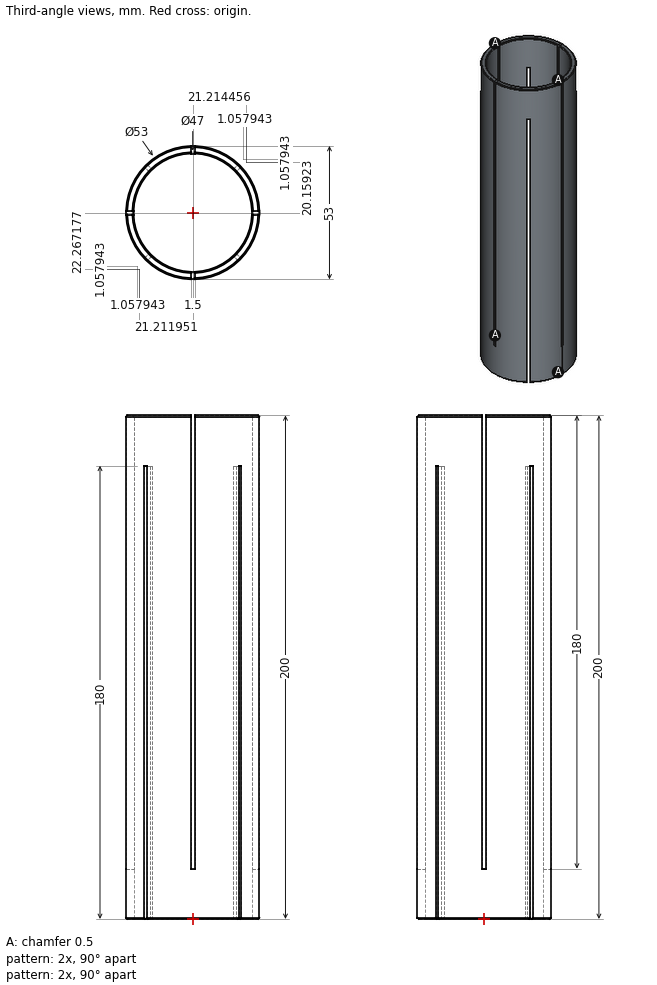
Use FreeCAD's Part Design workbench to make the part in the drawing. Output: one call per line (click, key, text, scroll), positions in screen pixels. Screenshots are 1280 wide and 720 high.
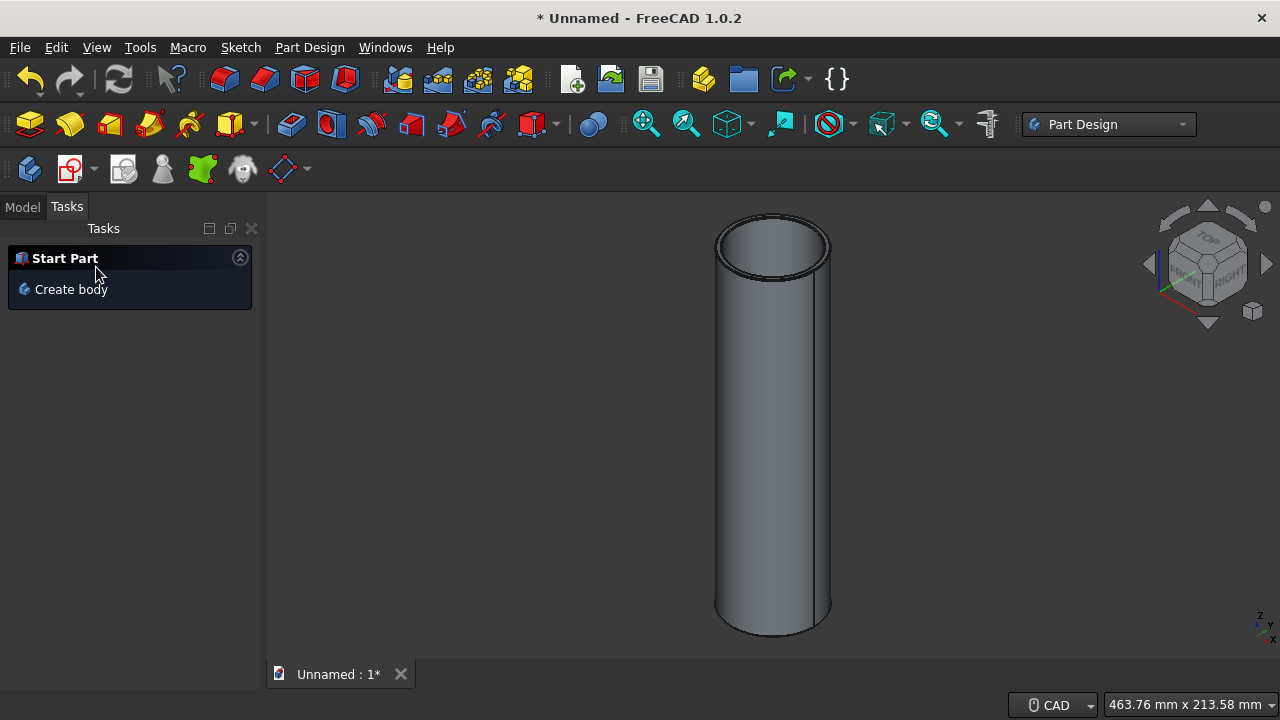
scroll(719, 238, up, 11)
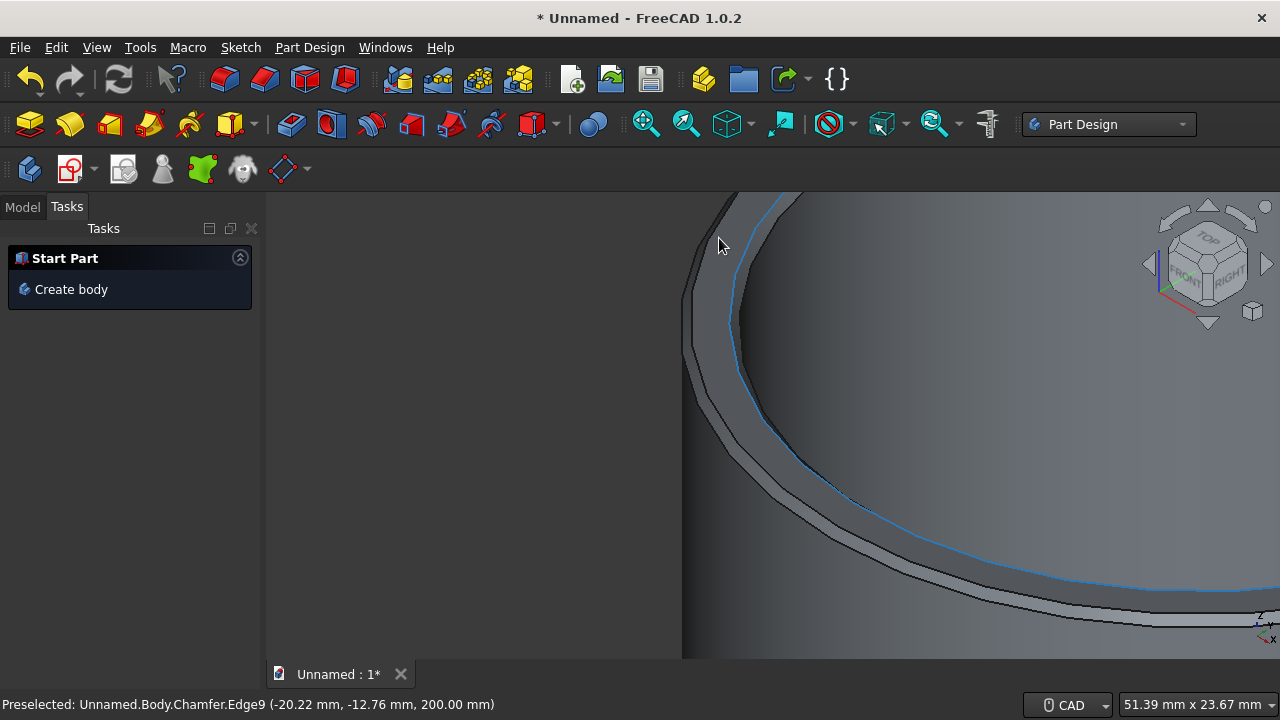
click(719, 245)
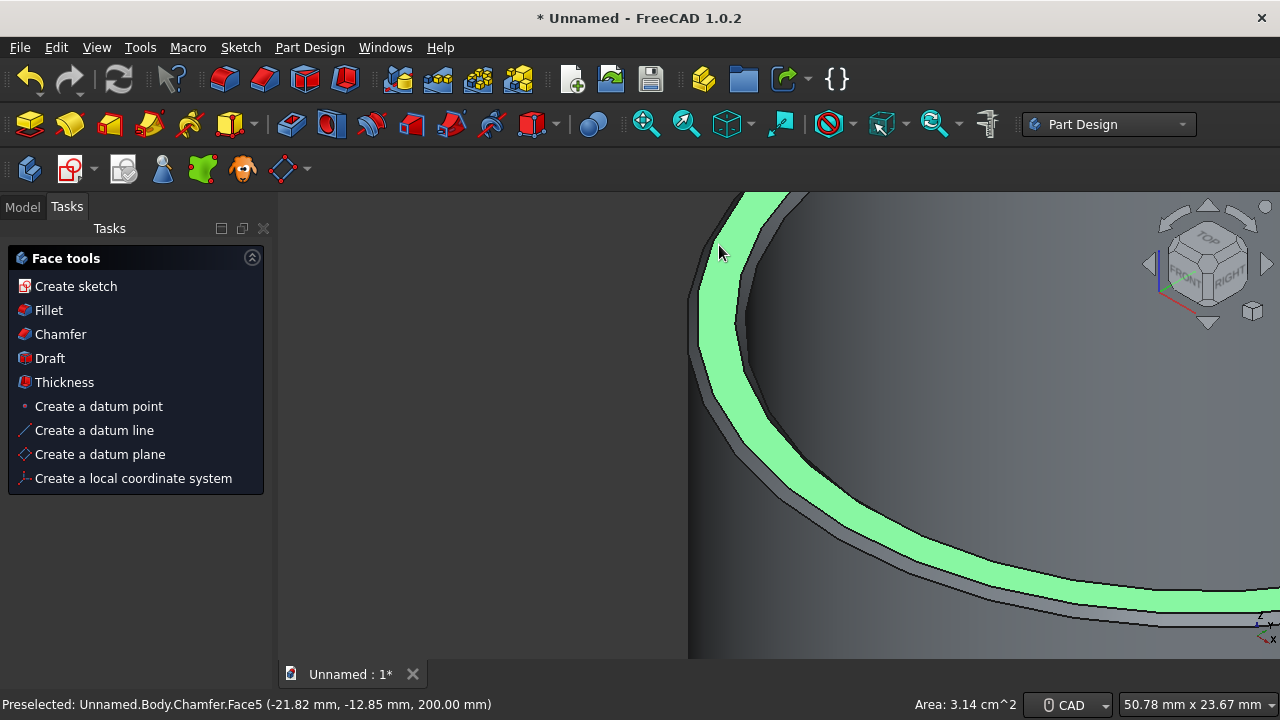
click(70, 170)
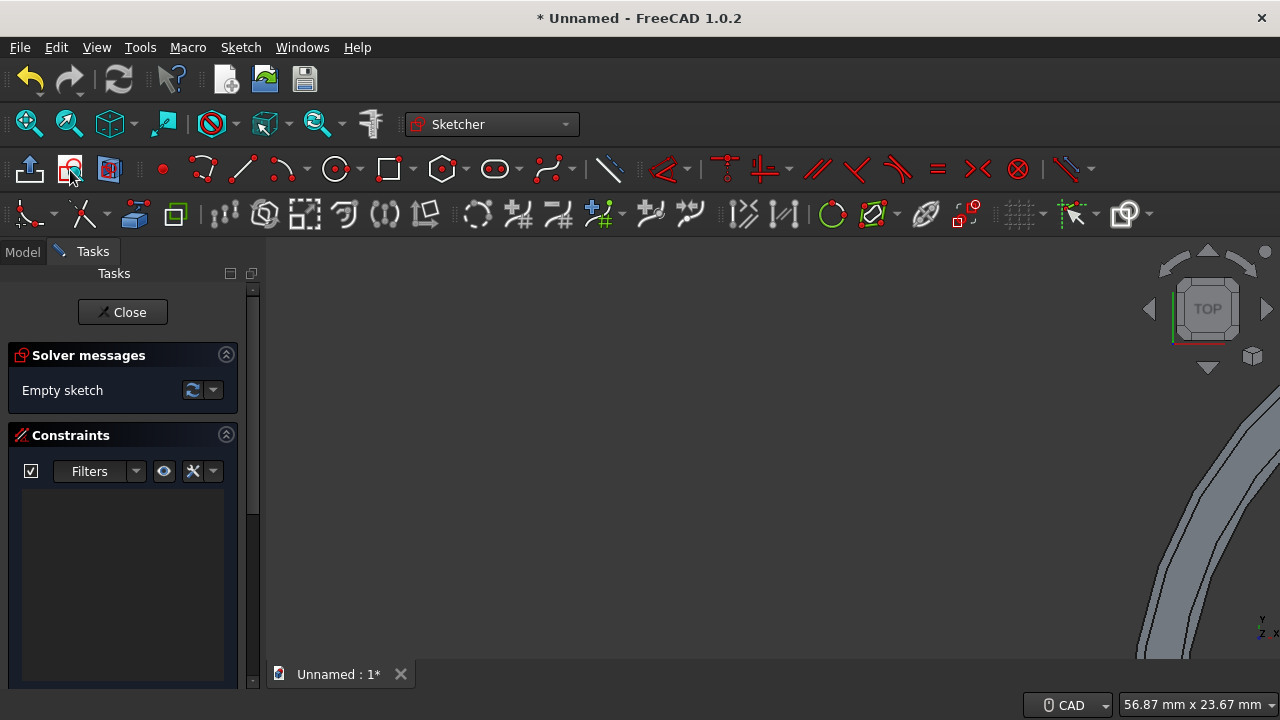
scroll(317, 327, down, 6)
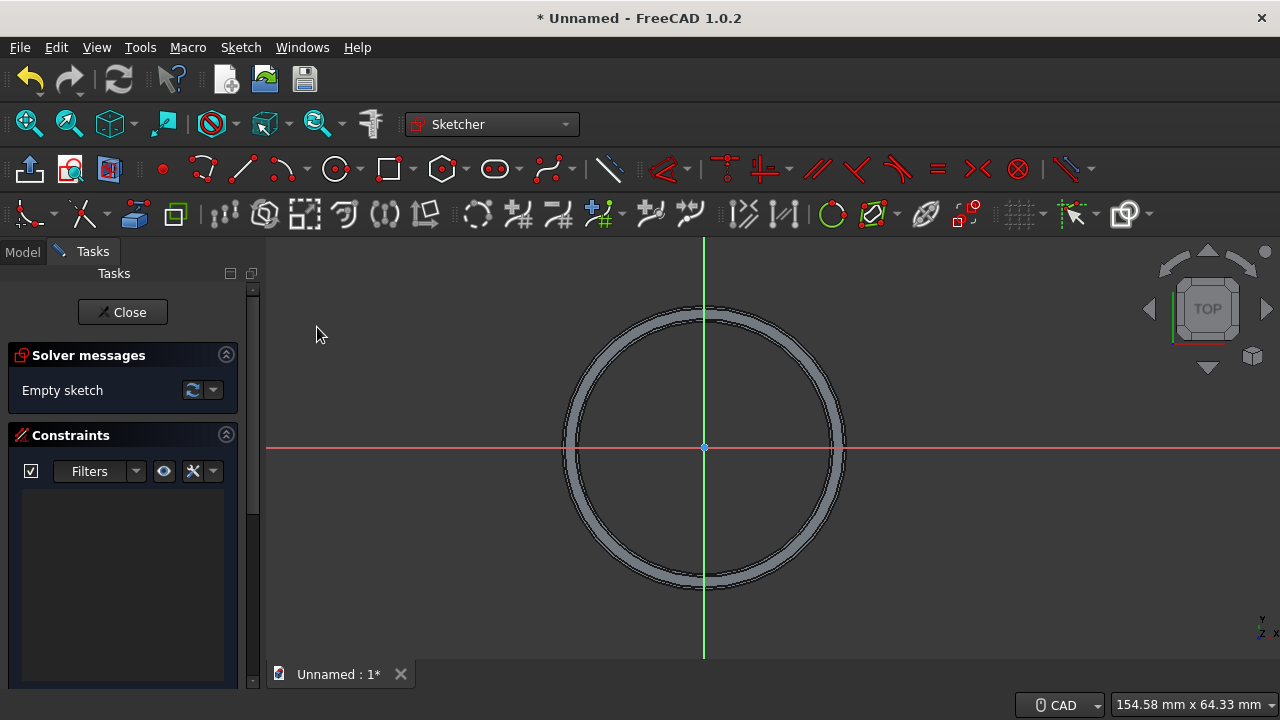
key(g)
key(v)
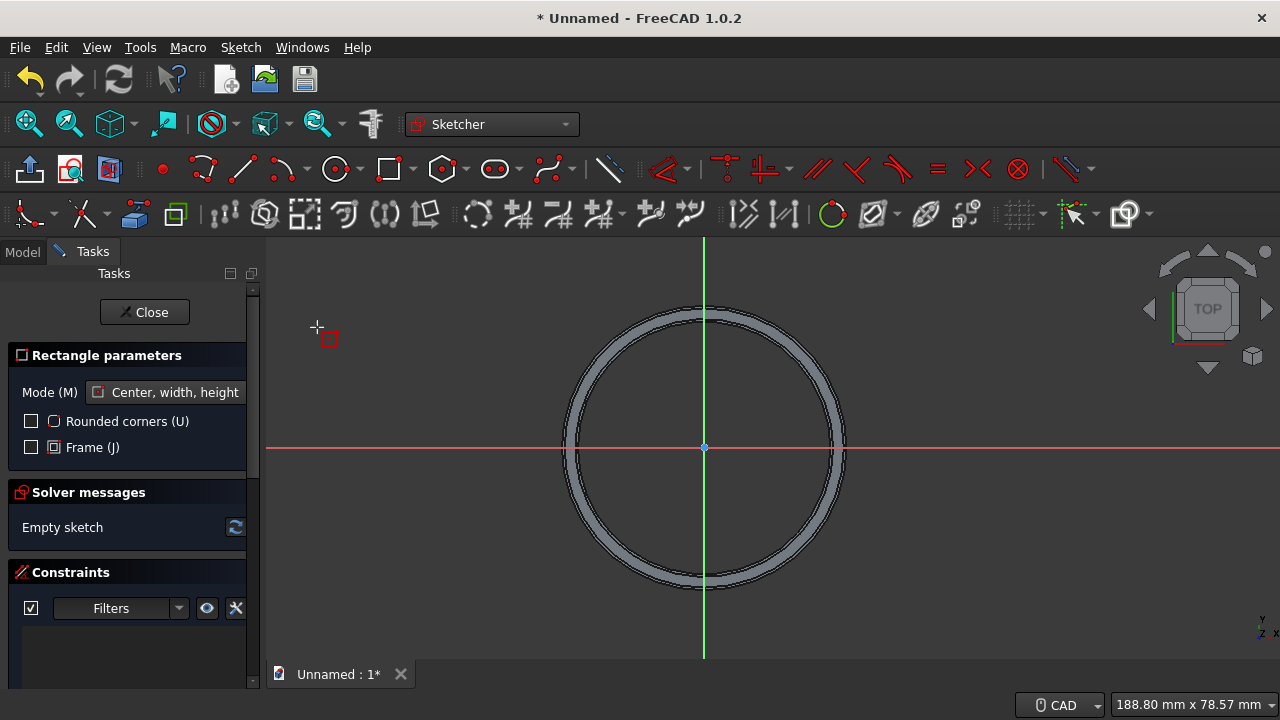
scroll(704, 448, up, 7)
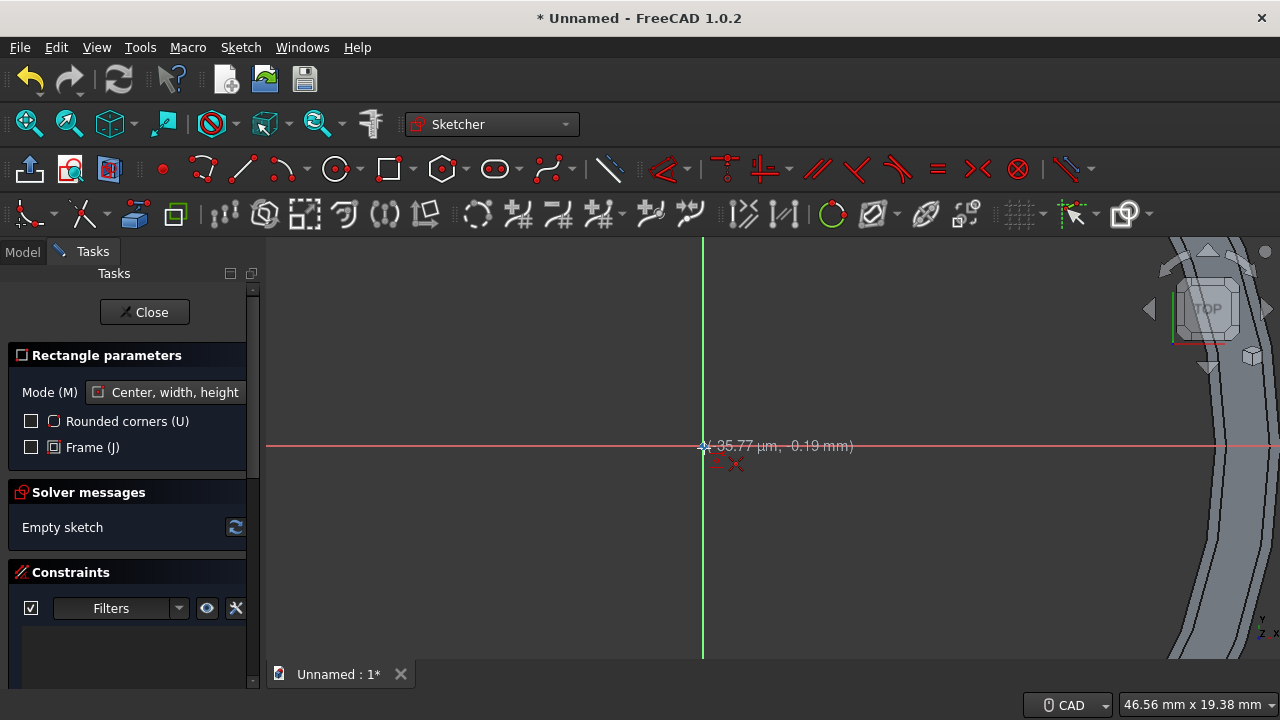
scroll(705, 449, down, 7)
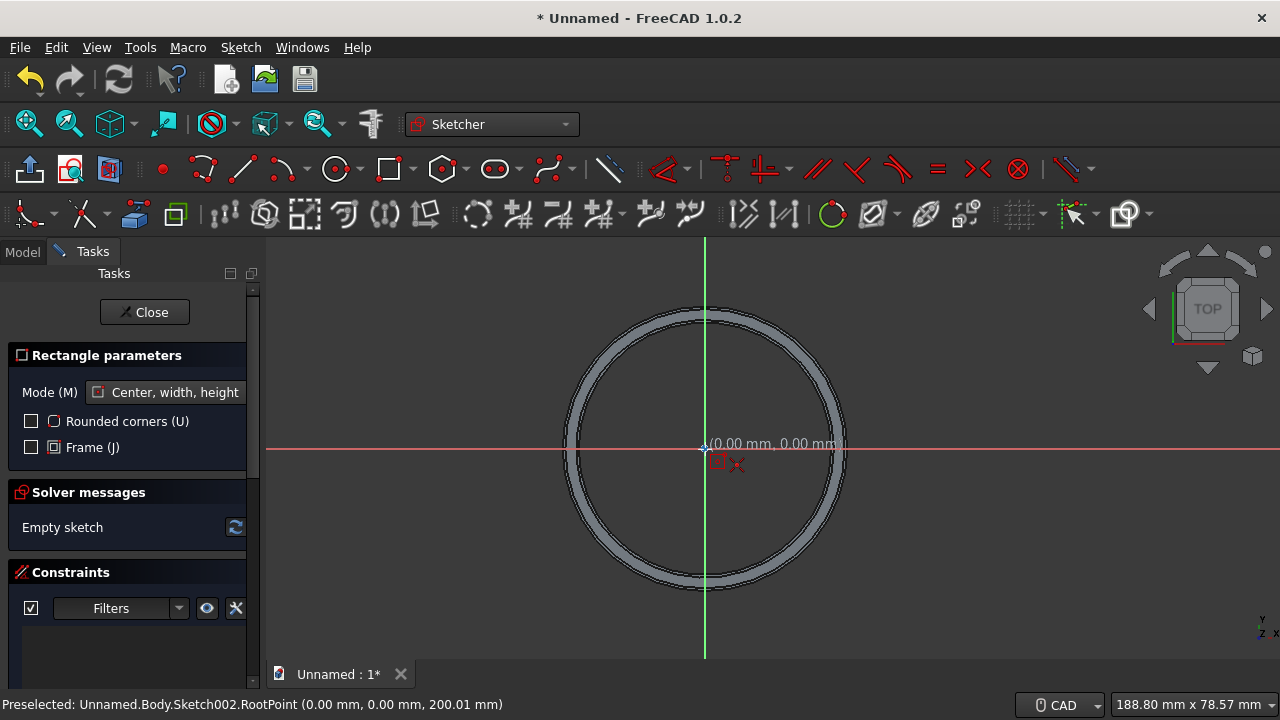
click(705, 449)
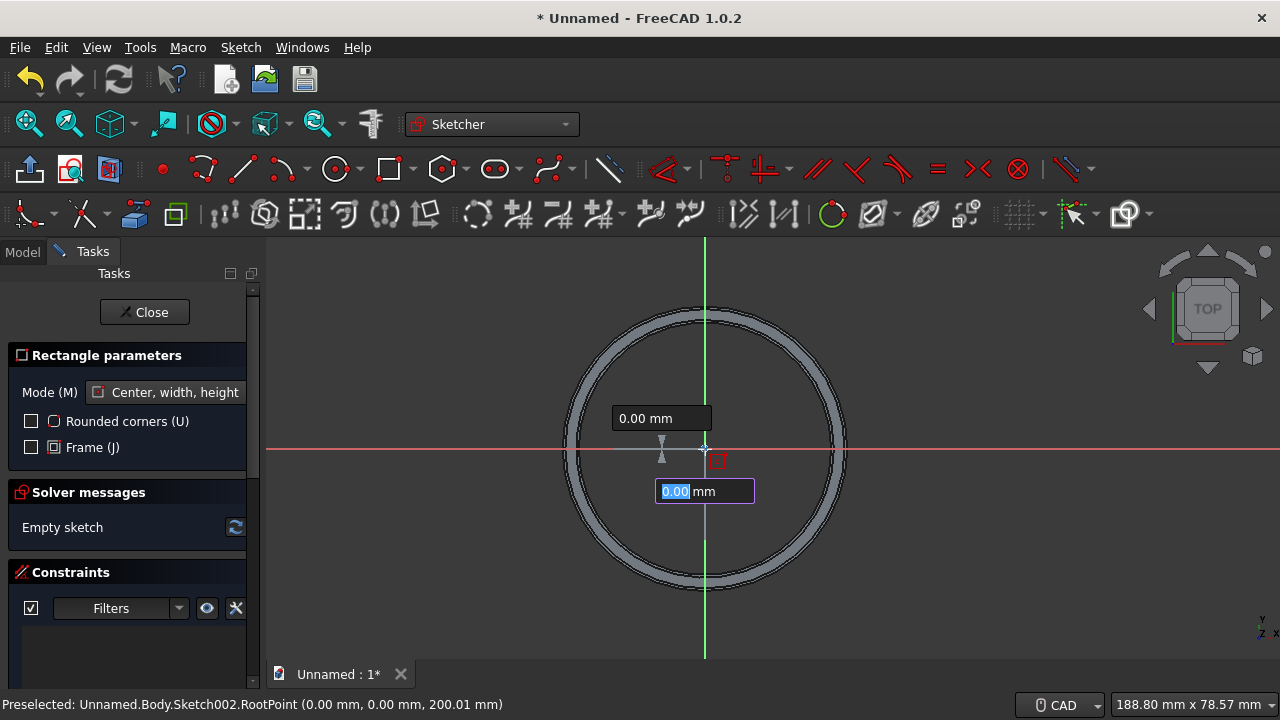
scroll(709, 306, up, 7)
move(708, 307)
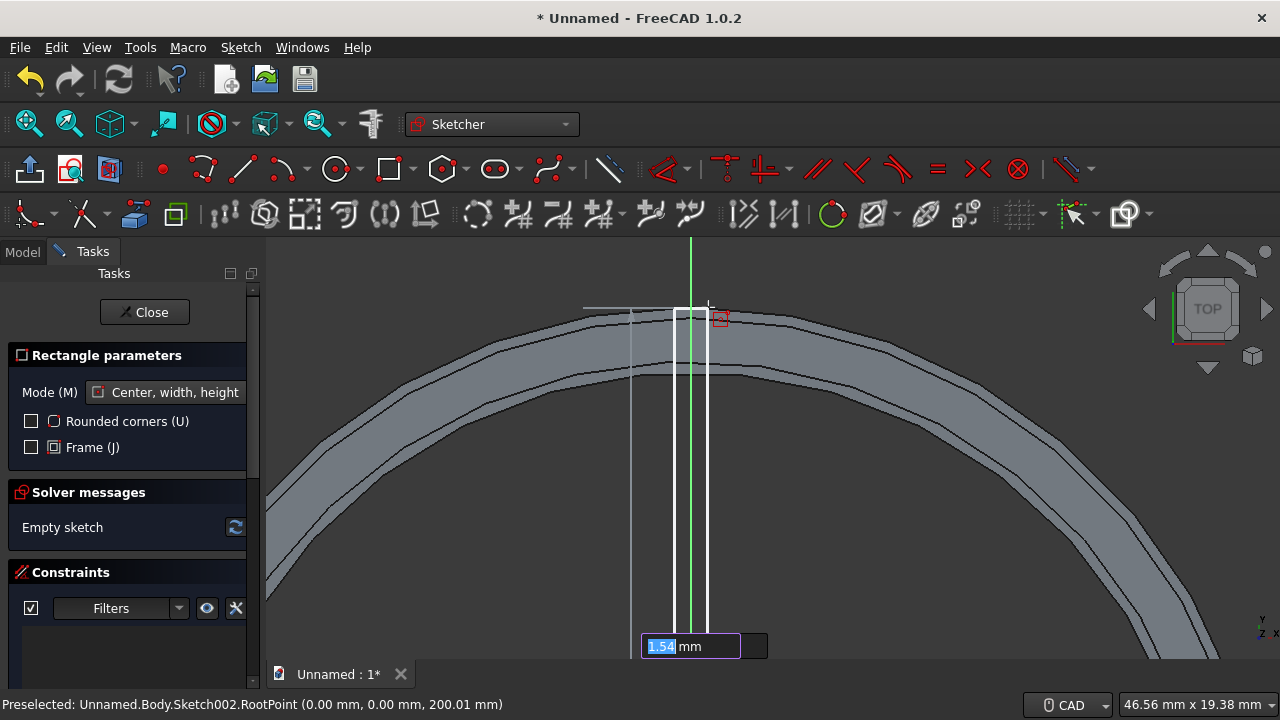
text(1.5)
key(Tab)
text(53)
key(Return)
key(Escape)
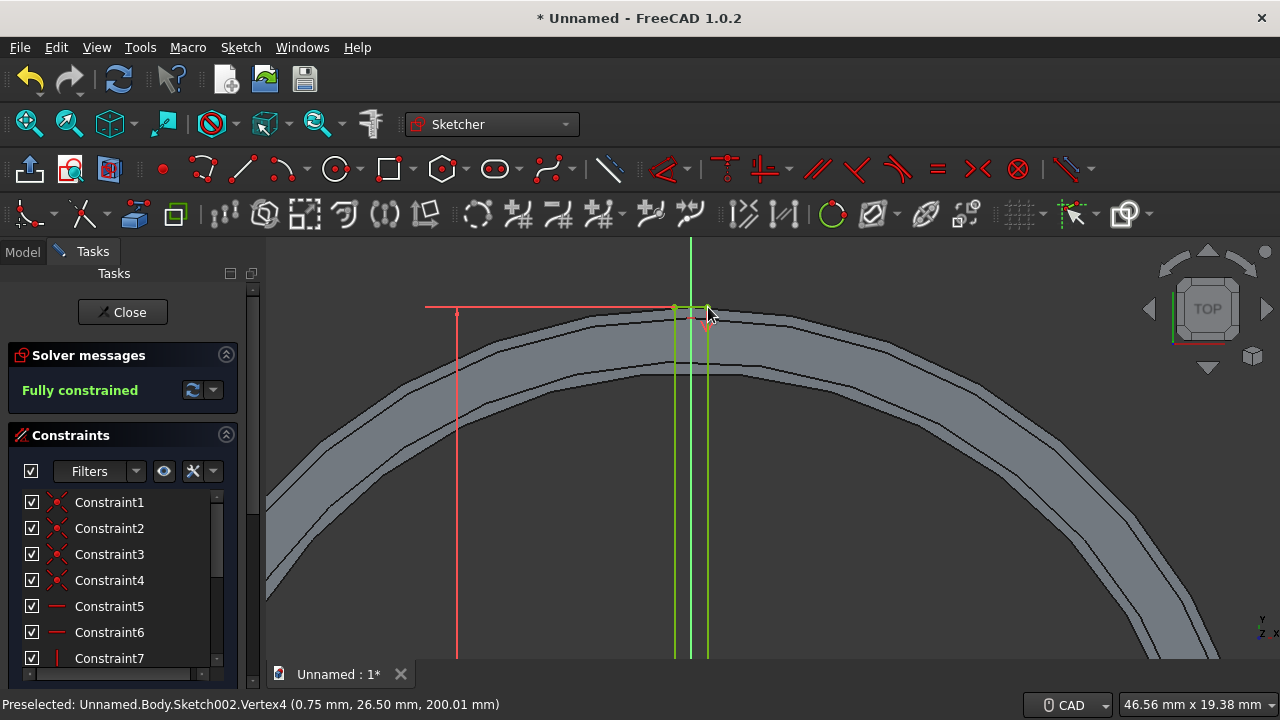
click(123, 312)